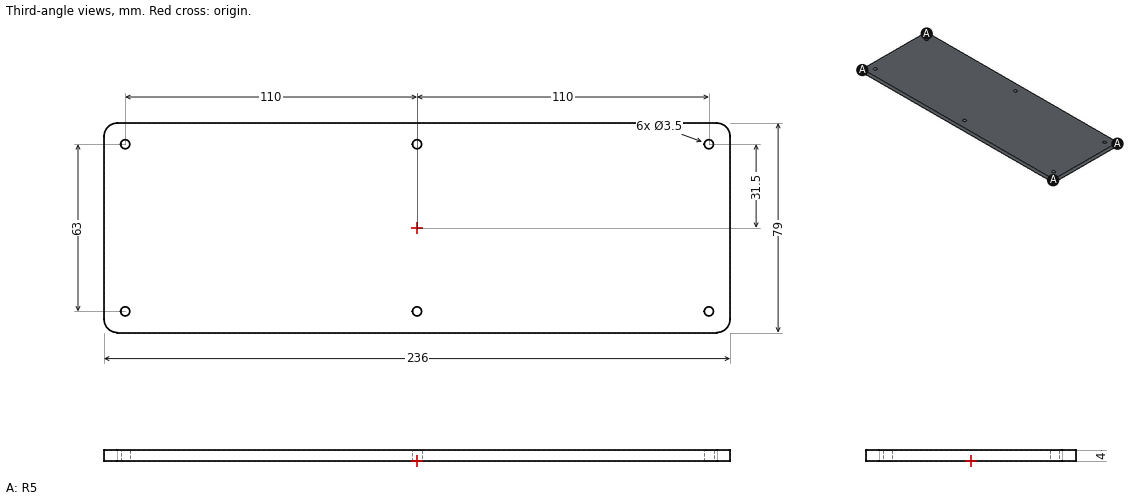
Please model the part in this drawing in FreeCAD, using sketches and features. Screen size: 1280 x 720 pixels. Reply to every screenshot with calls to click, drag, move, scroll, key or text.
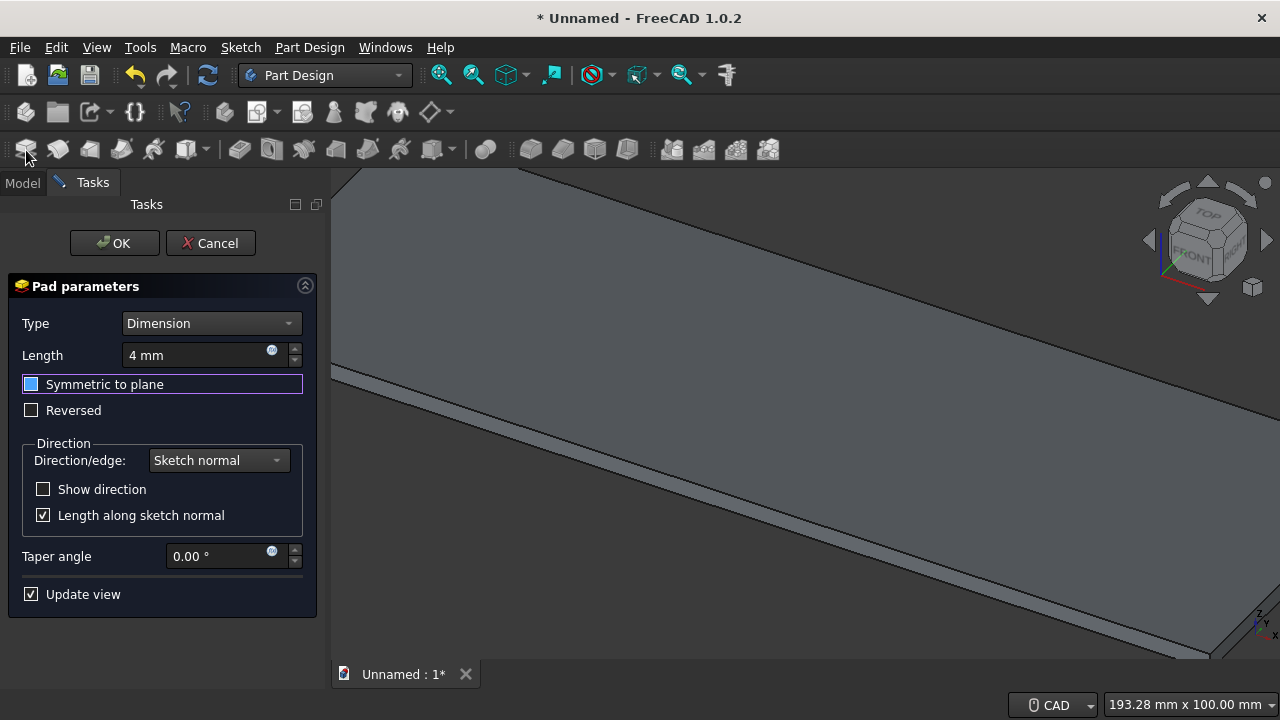
click(115, 243)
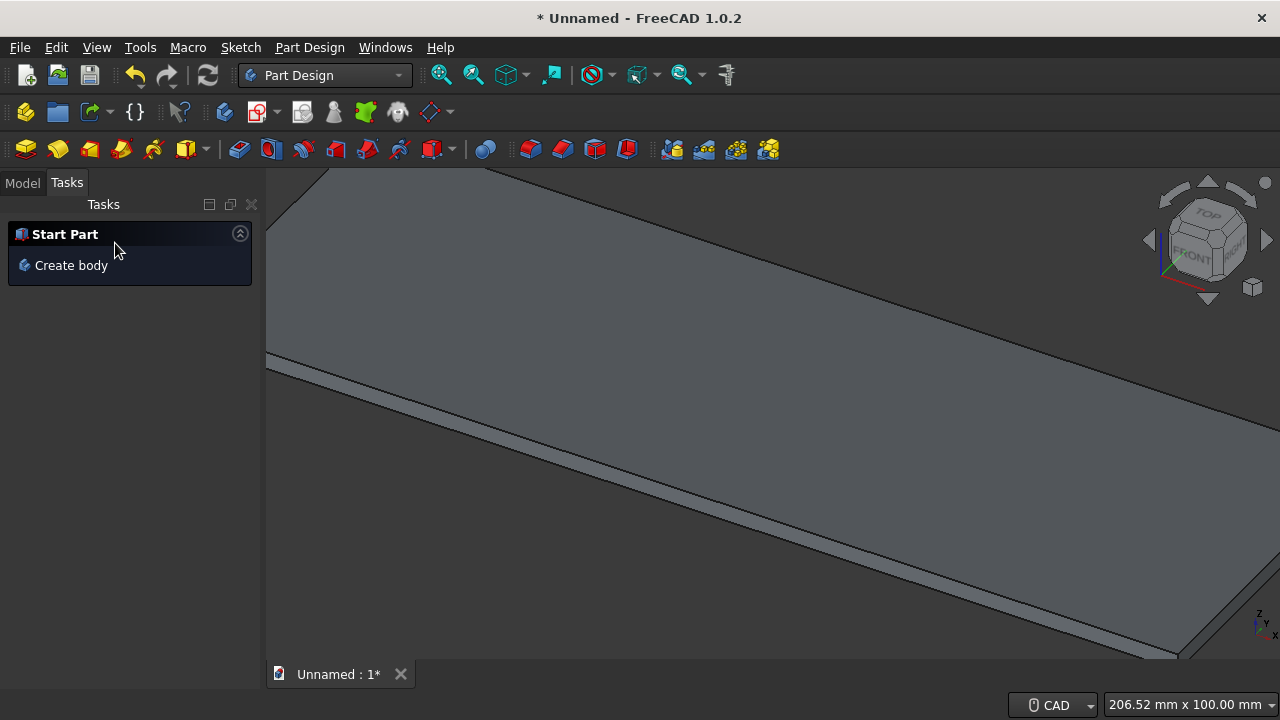
click(442, 76)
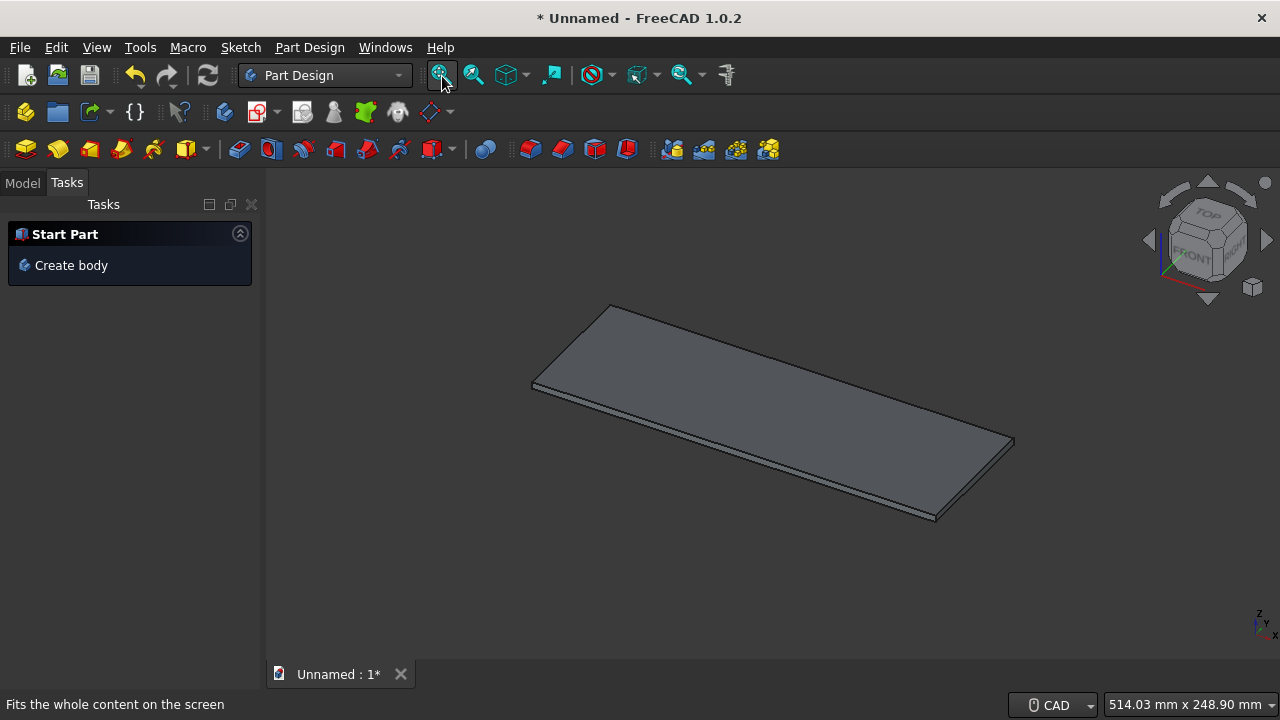
scroll(610, 307, up, 9)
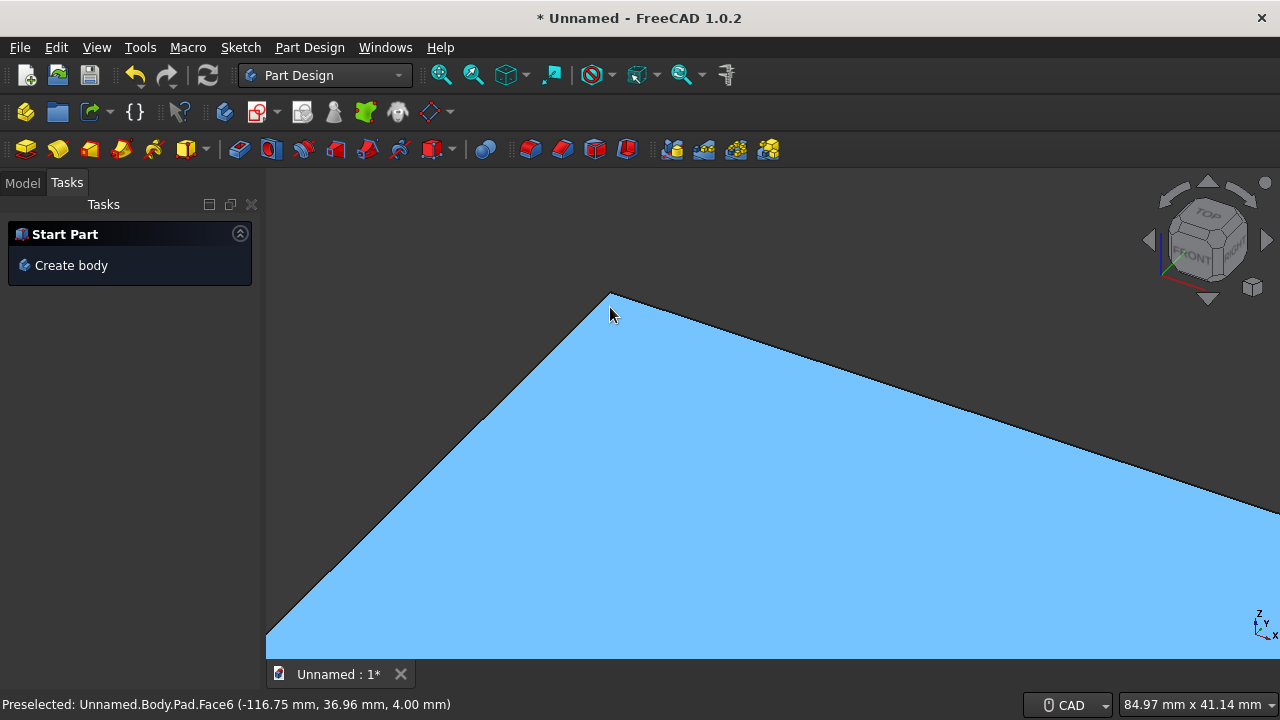
click(442, 76)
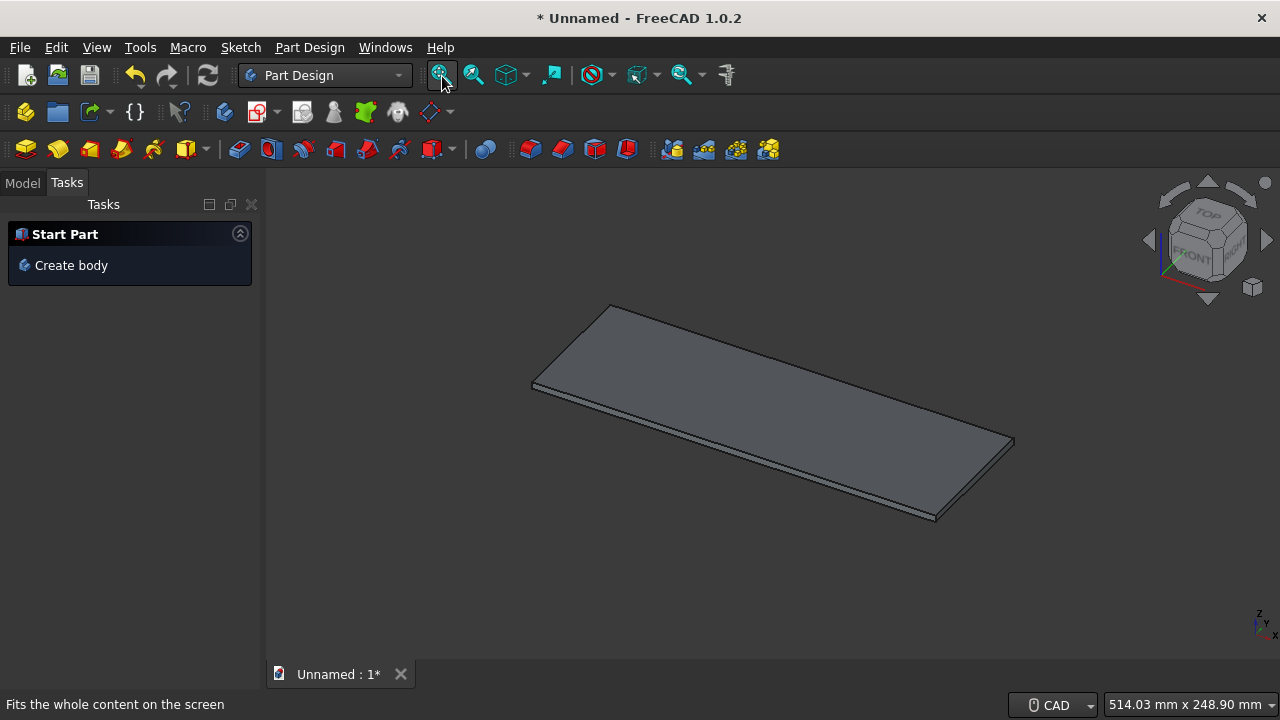
key(0)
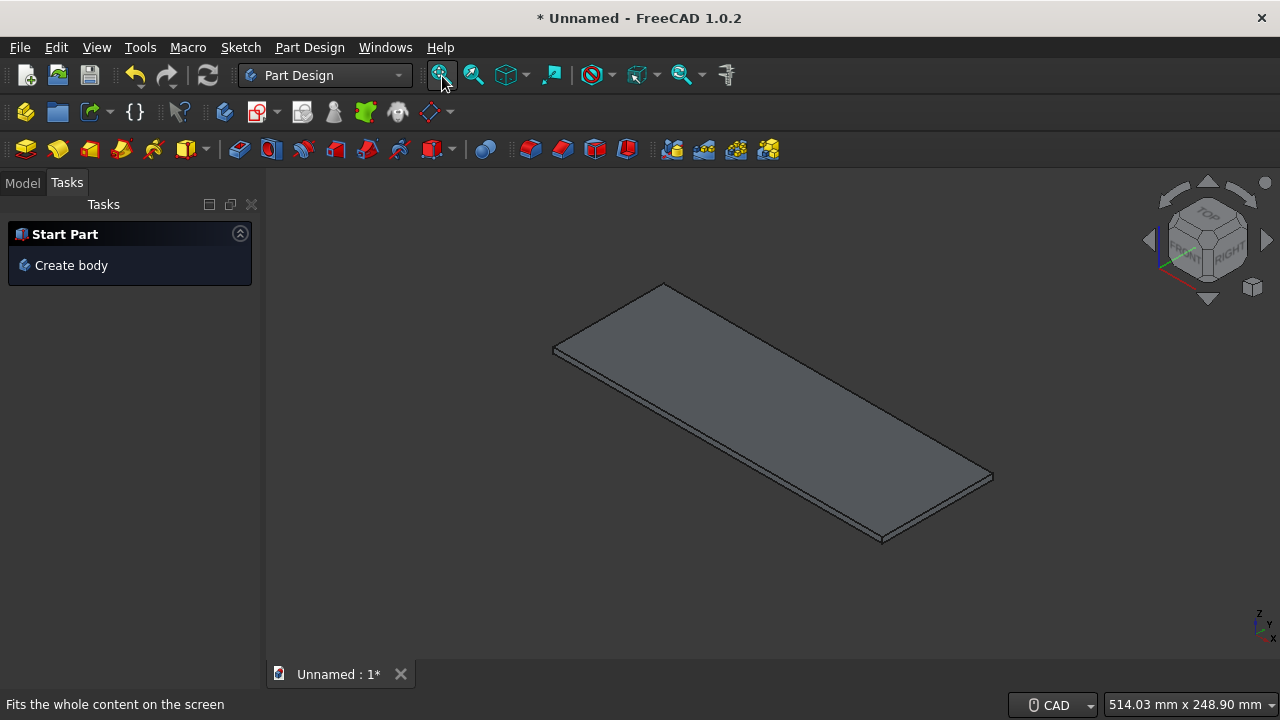
scroll(664, 286, up, 9)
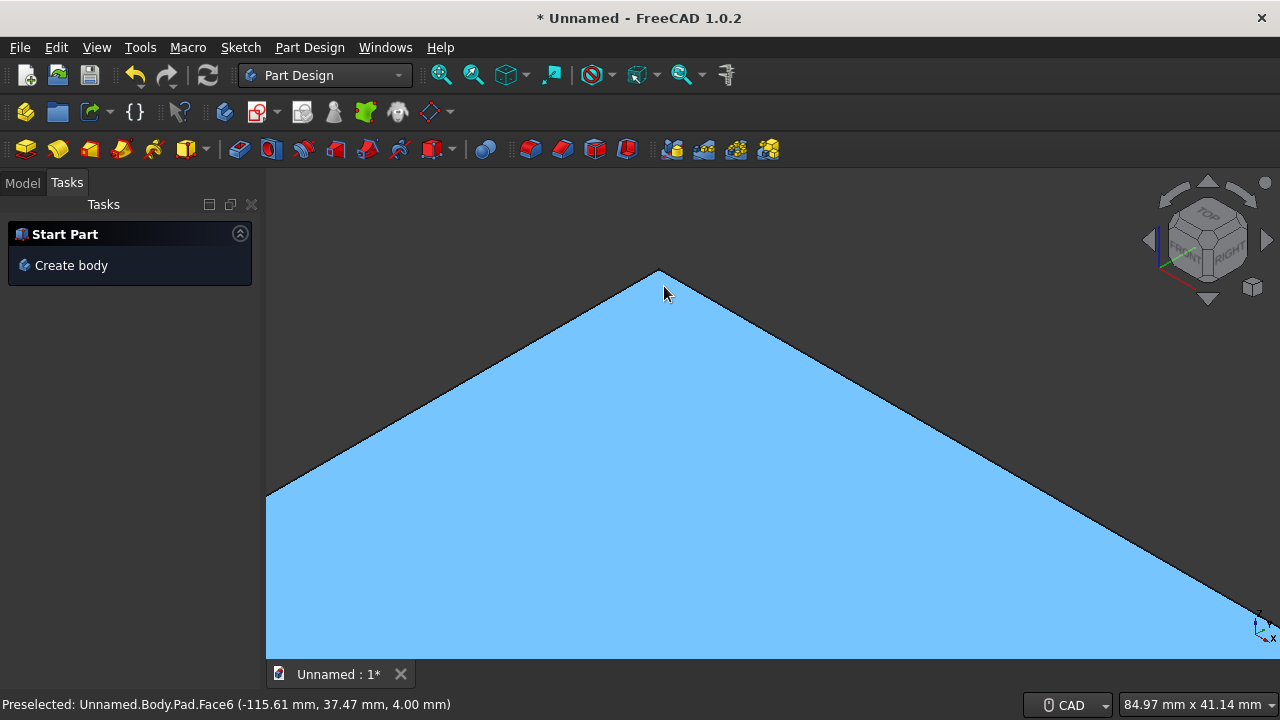
click(442, 76)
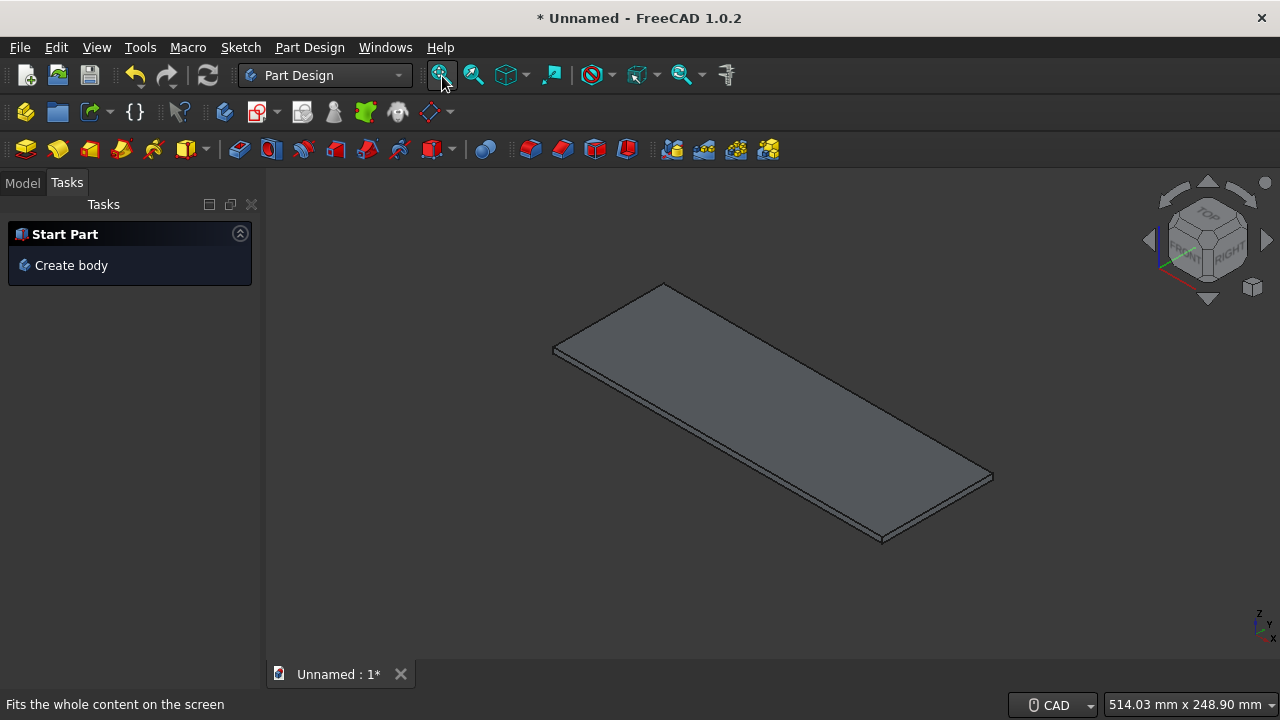
key(2)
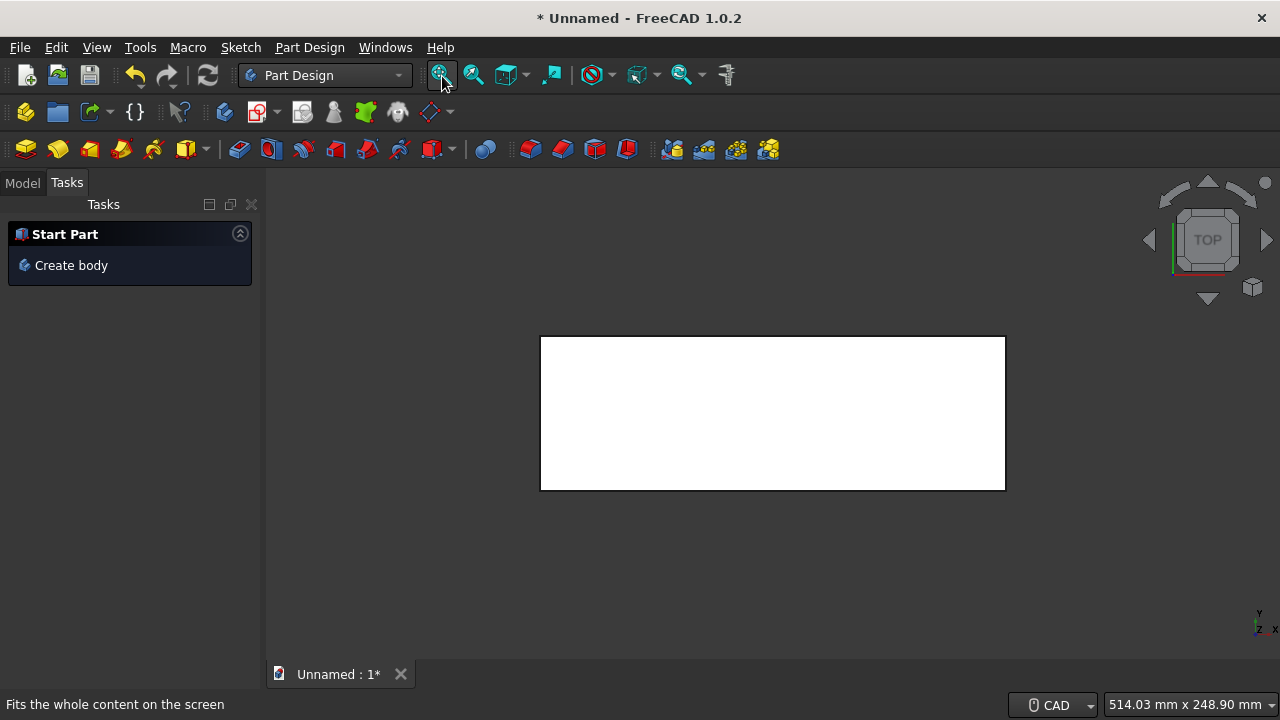
scroll(540, 335, up, 9)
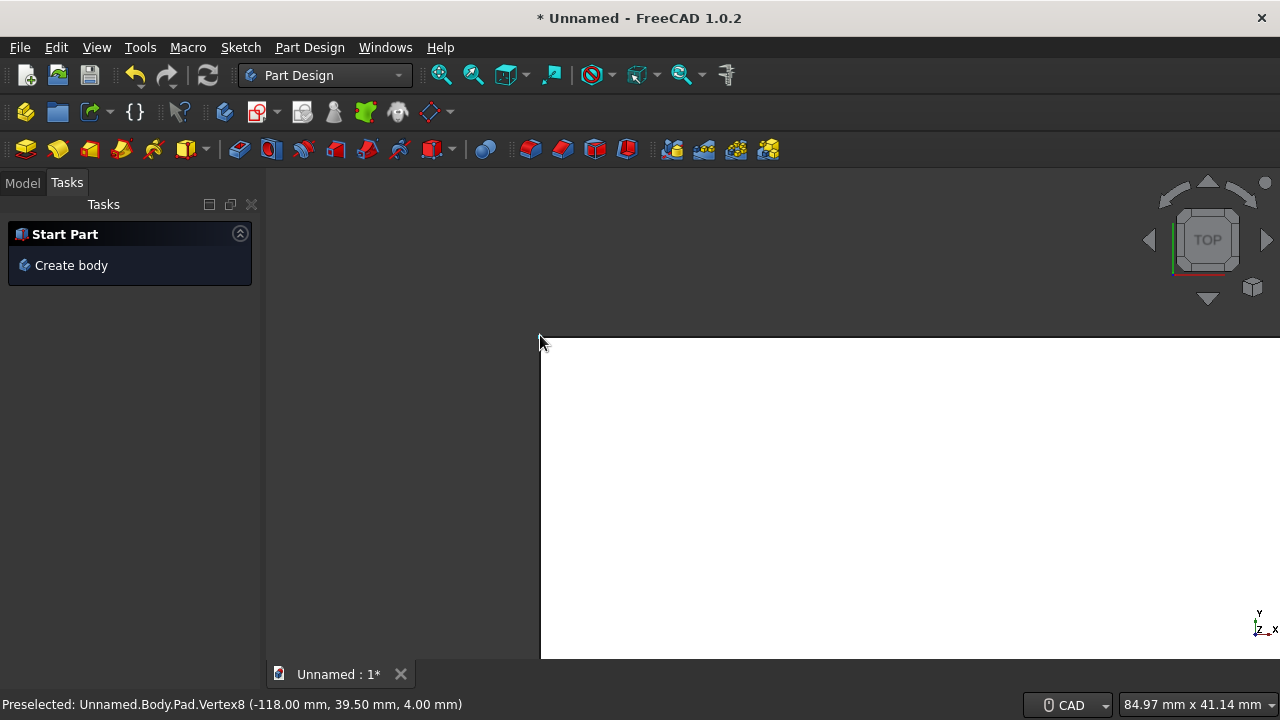
click(442, 76)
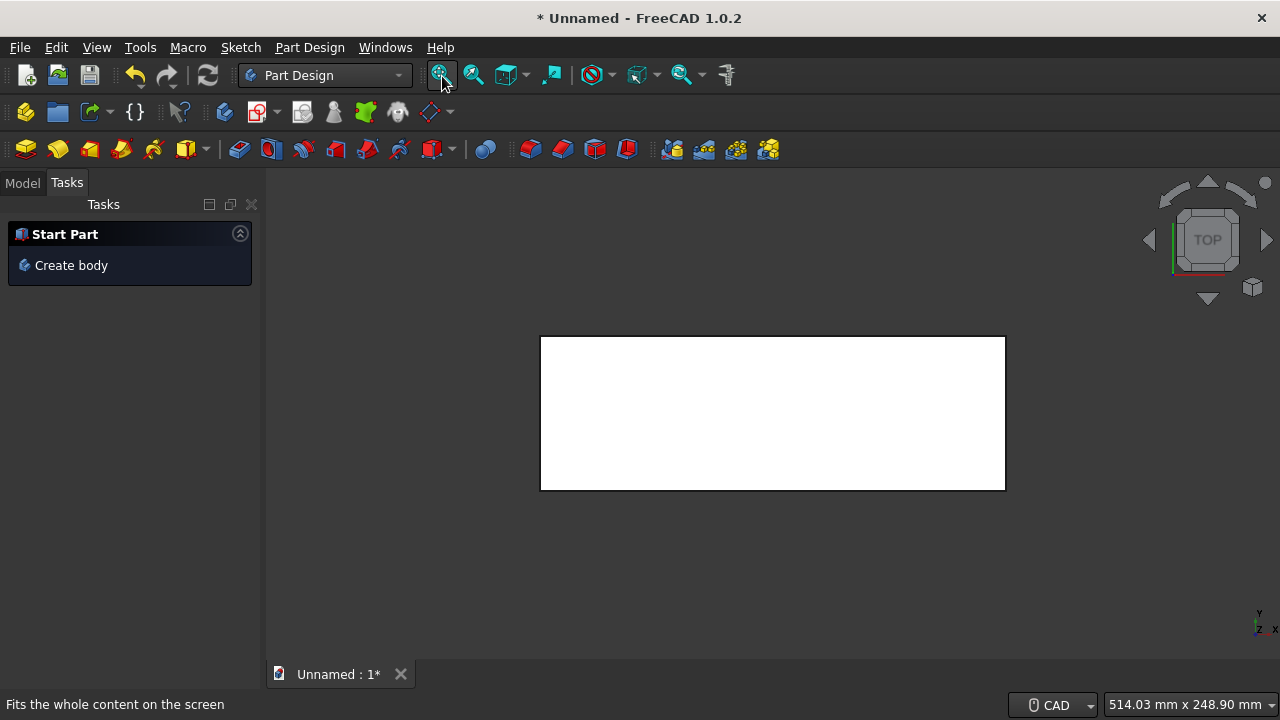
key(1)